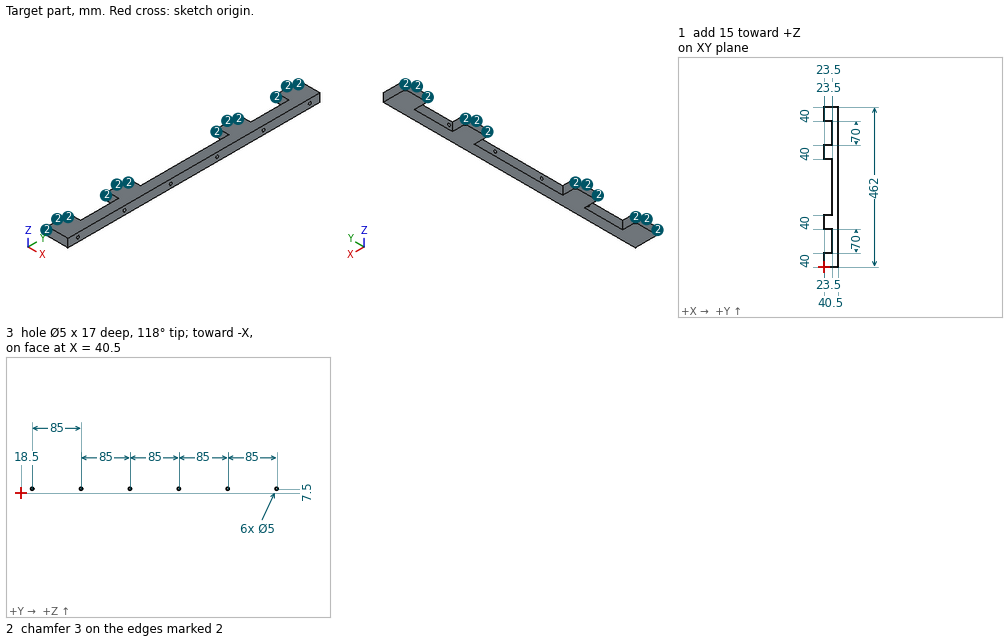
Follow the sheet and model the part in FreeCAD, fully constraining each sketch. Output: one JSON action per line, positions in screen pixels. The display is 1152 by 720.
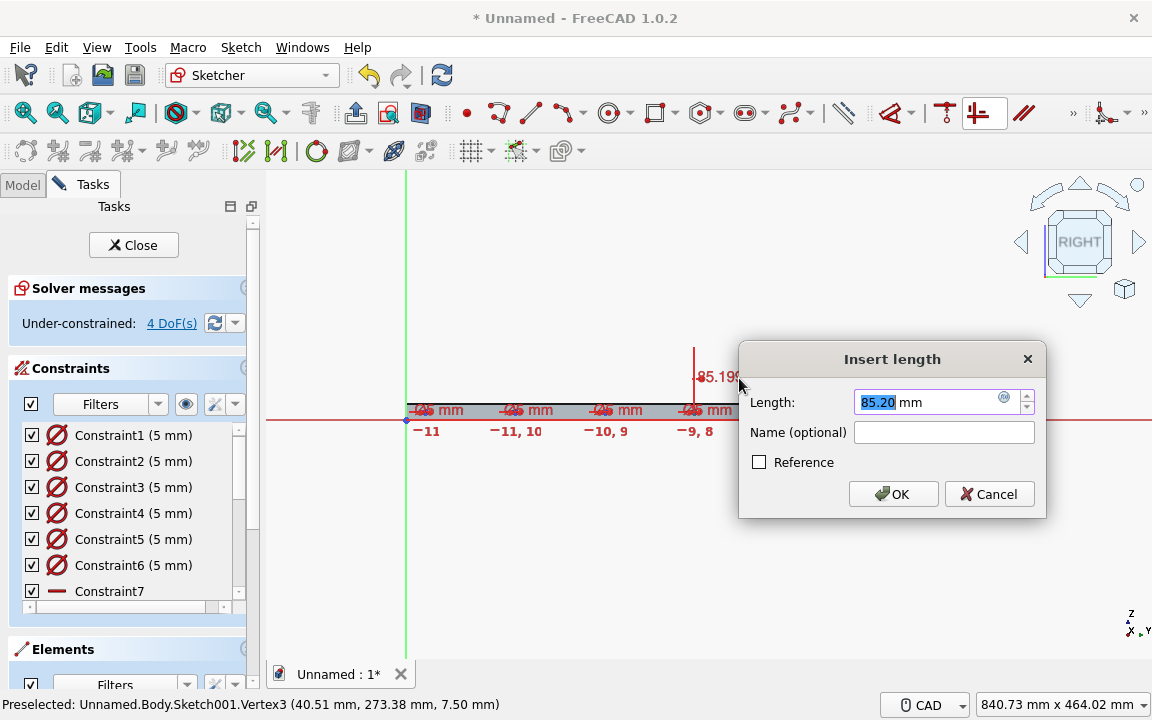
{"action": "type", "text": "85"}
{"action": "key", "text": "Return"}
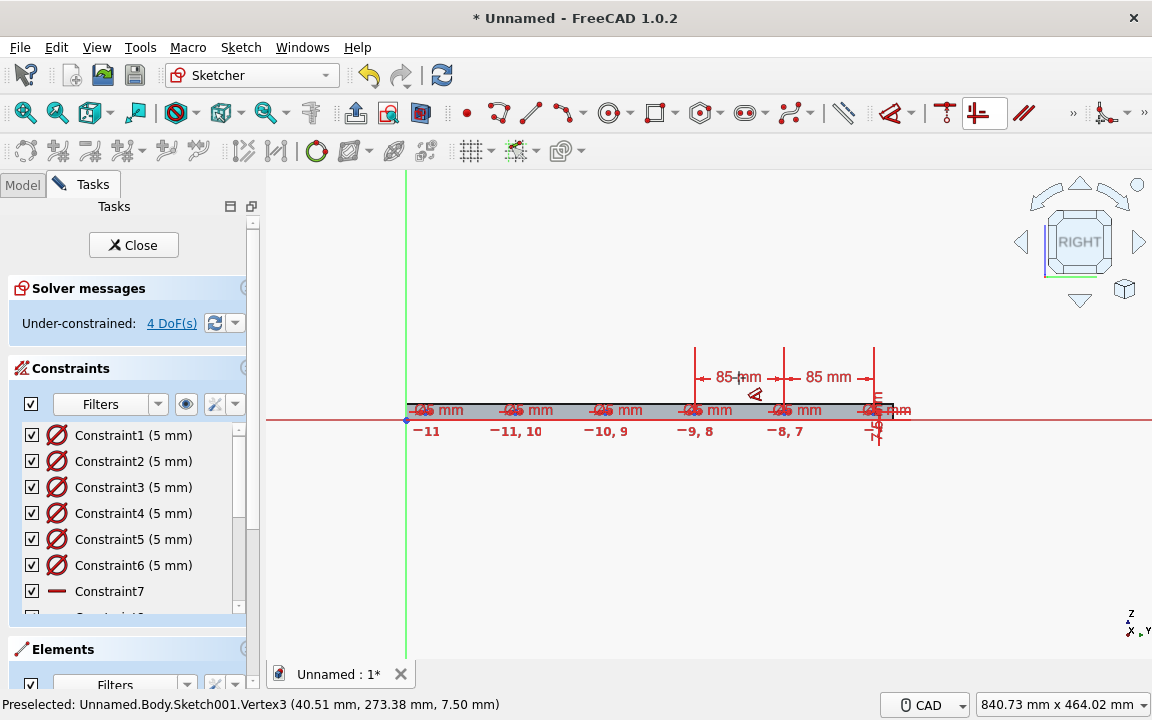
{"action": "left_click", "coordinate": [695, 412]}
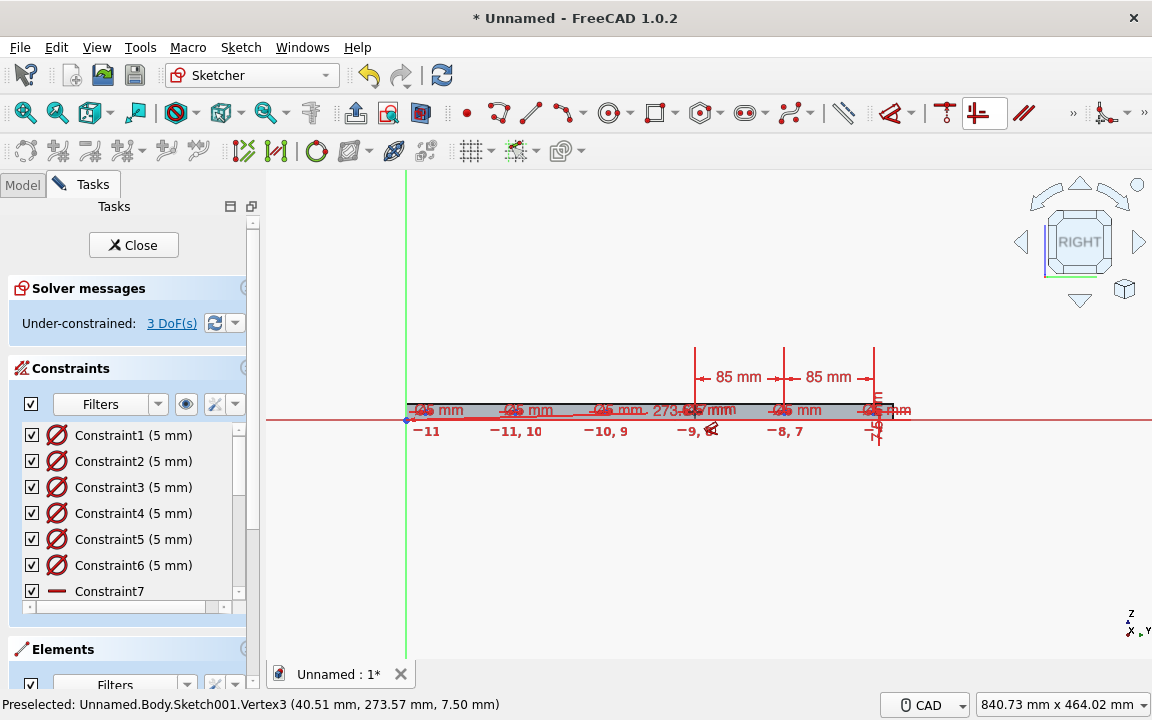
{"action": "left_click", "coordinate": [605, 412]}
{"action": "left_click", "coordinate": [650, 378]}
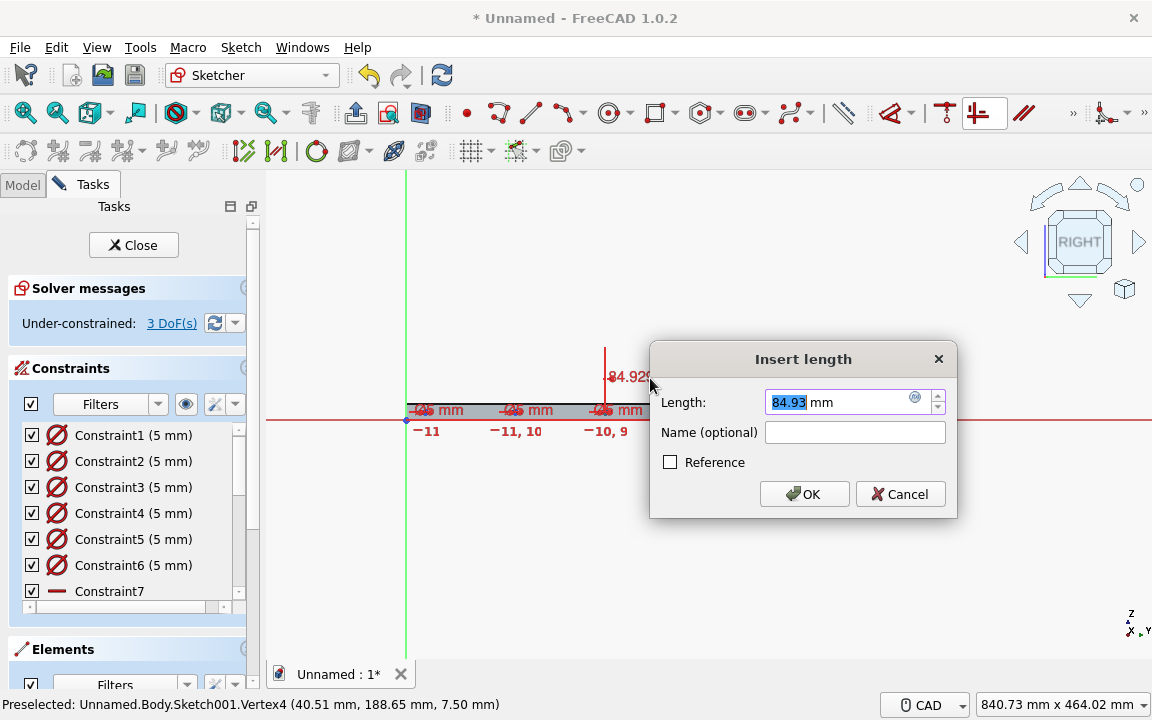
{"action": "type", "text": "85"}
{"action": "key", "text": "Return"}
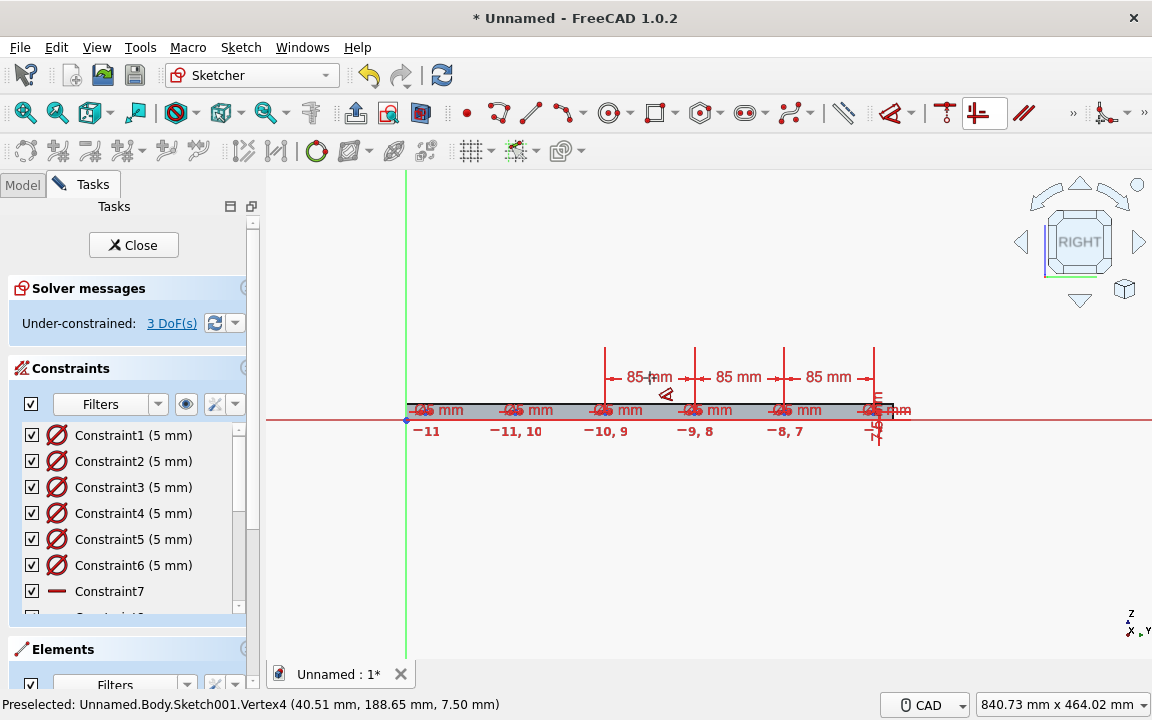
{"action": "left_click", "coordinate": [605, 412]}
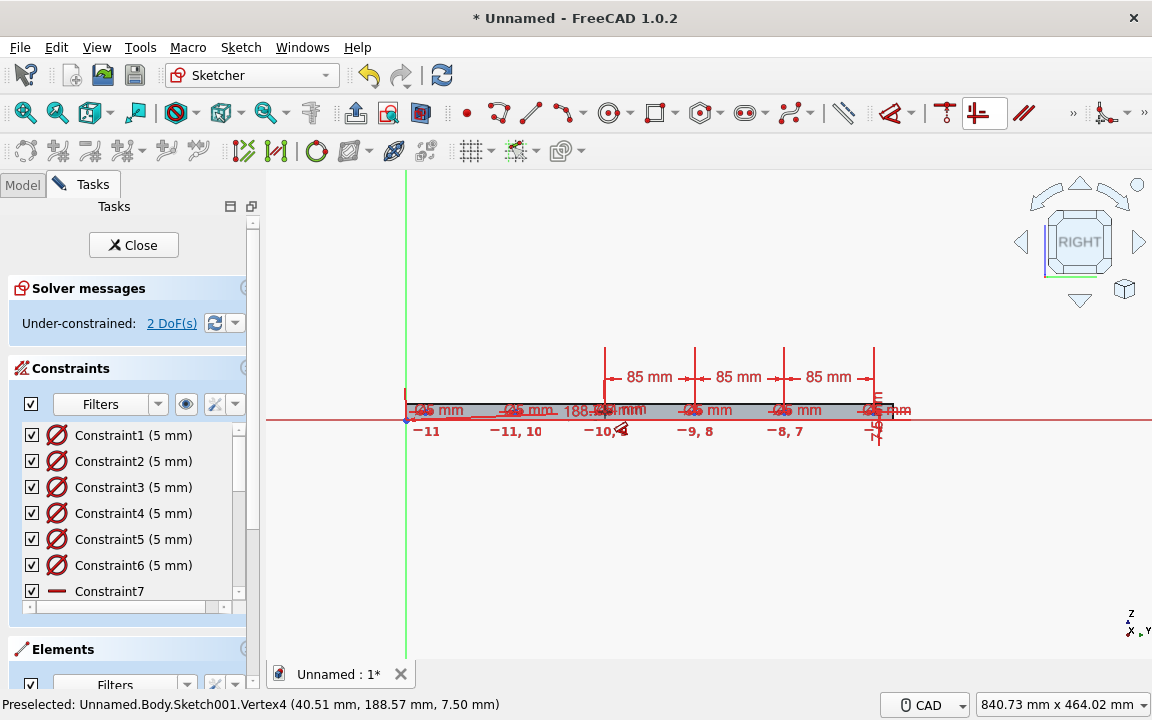
{"action": "left_click", "coordinate": [515, 412]}
{"action": "left_click", "coordinate": [560, 378]}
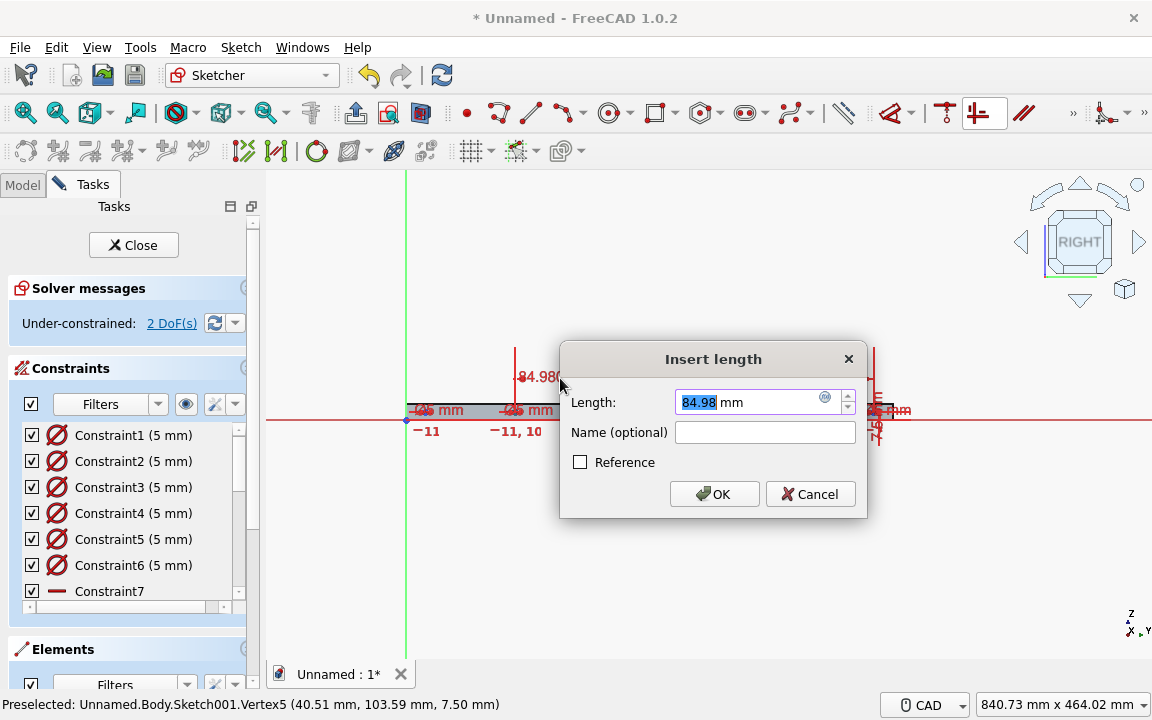
{"action": "type", "text": "85"}
{"action": "key", "text": "Return"}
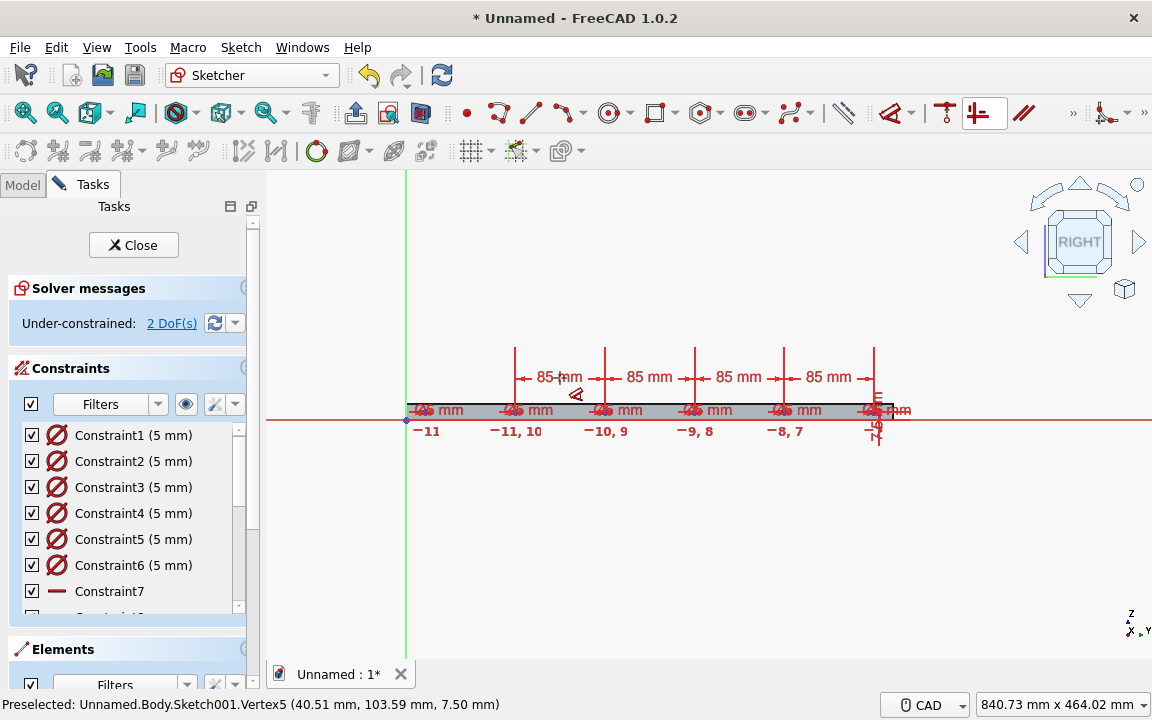
{"action": "left_click", "coordinate": [515, 412]}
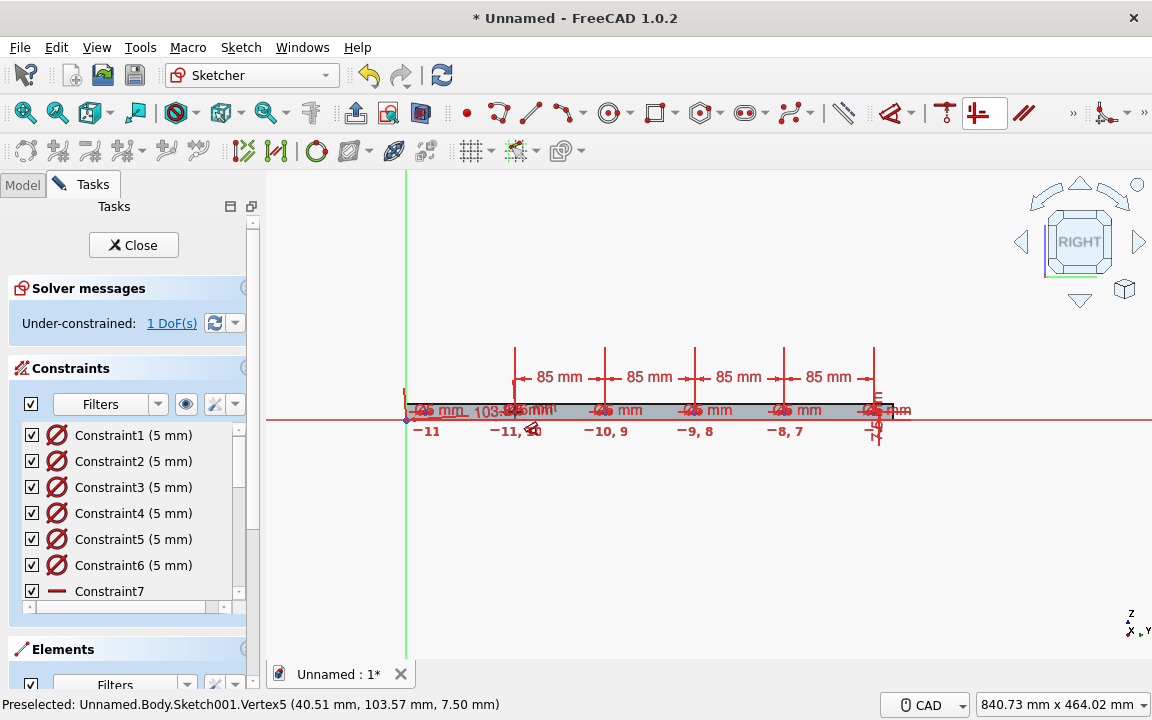
{"action": "left_click", "coordinate": [426, 412]}
{"action": "left_click", "coordinate": [471, 378]}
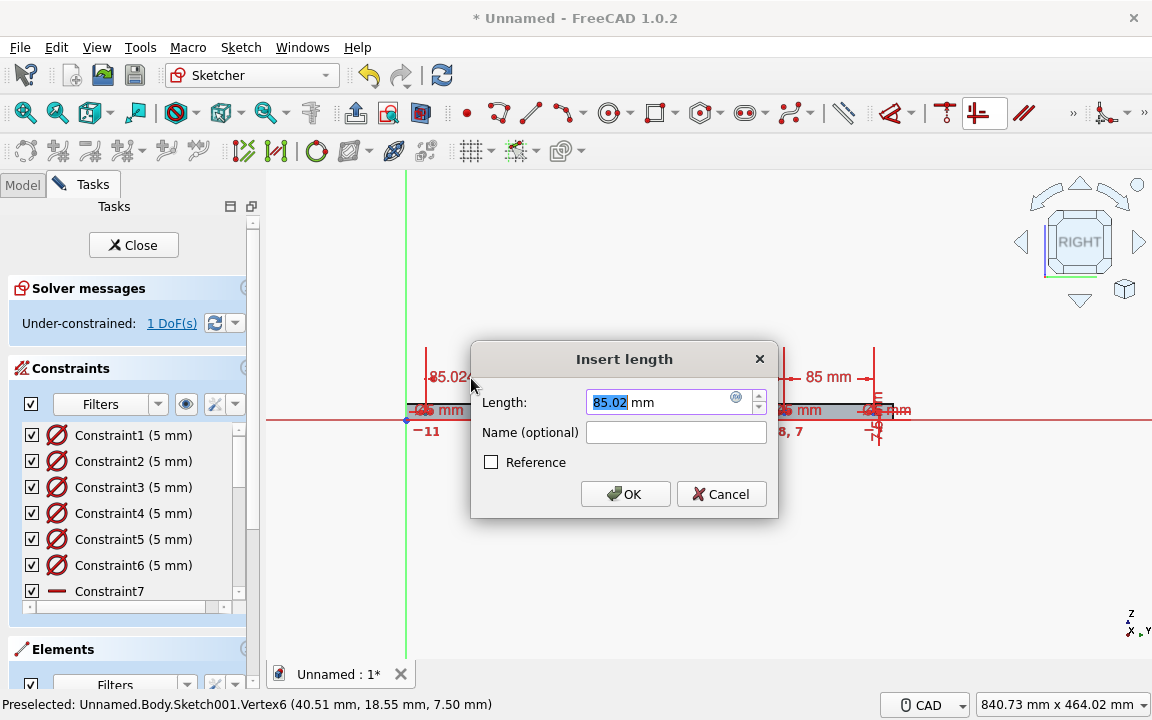
{"action": "type", "text": "85"}
{"action": "key", "text": "Return"}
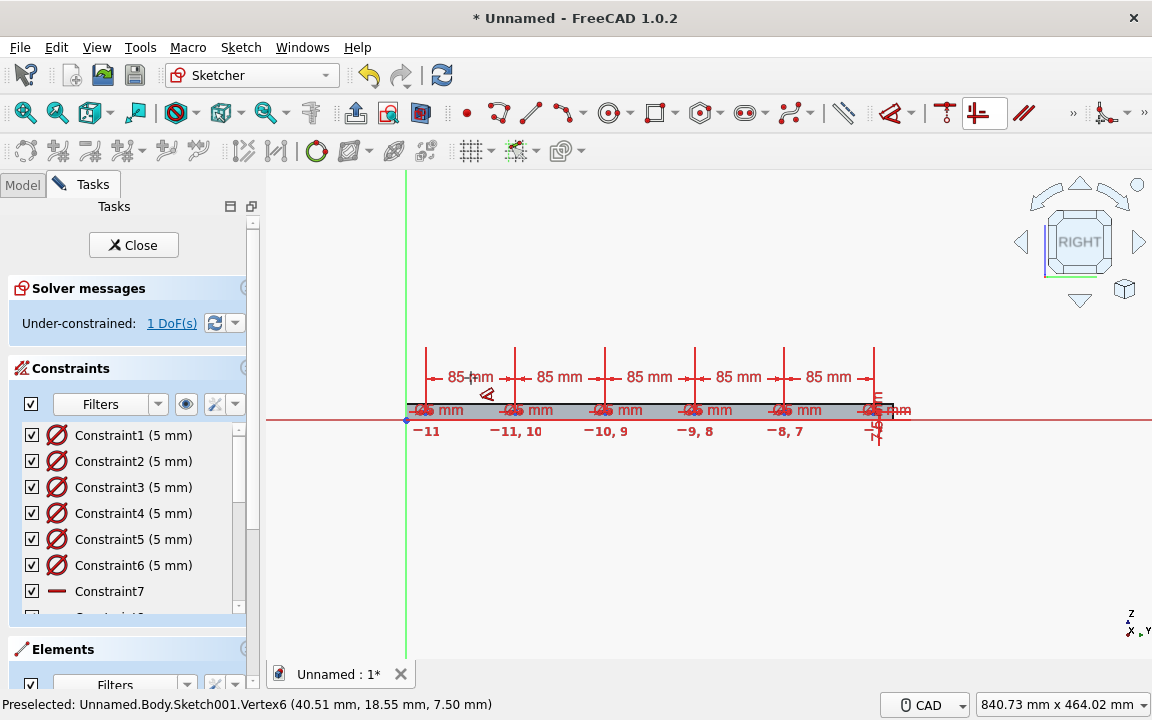
{"action": "scroll", "coordinate": [426, 412], "scroll_direction": "up", "scroll_amount": 4}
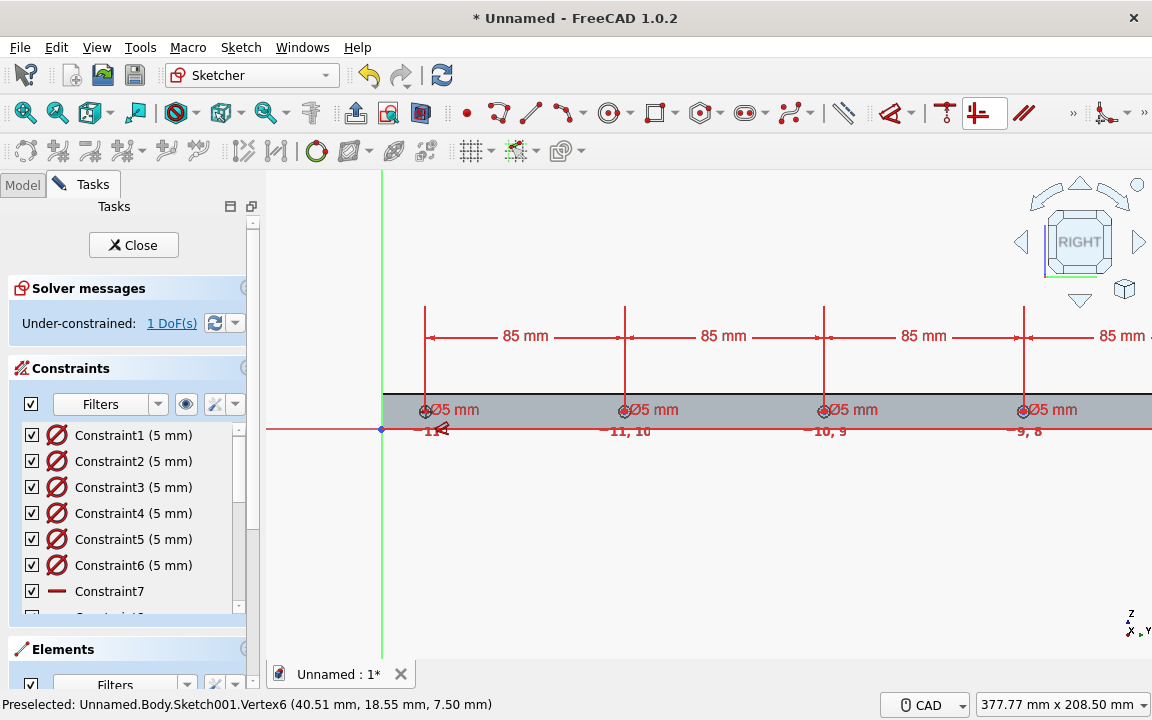
{"action": "left_click", "coordinate": [425, 412]}
{"action": "left_click", "coordinate": [404, 463]}